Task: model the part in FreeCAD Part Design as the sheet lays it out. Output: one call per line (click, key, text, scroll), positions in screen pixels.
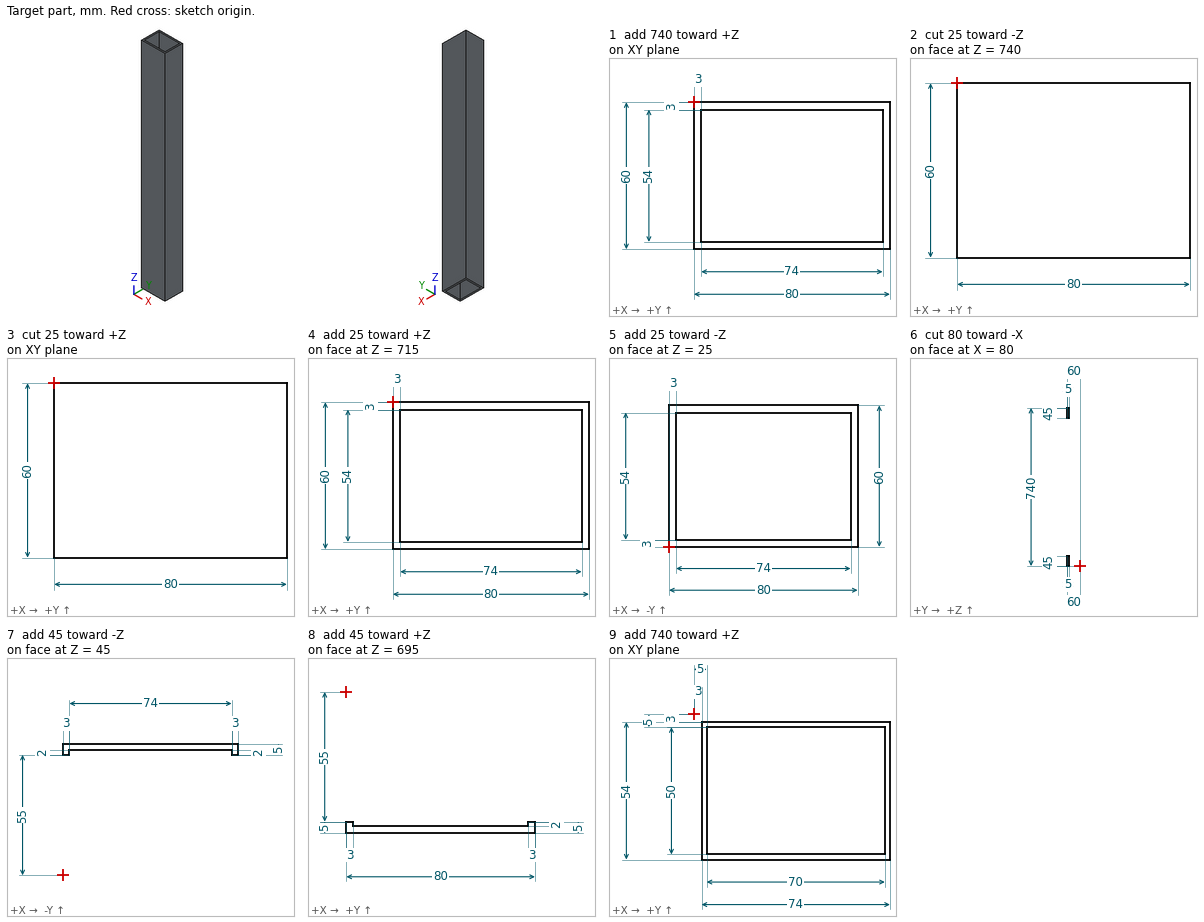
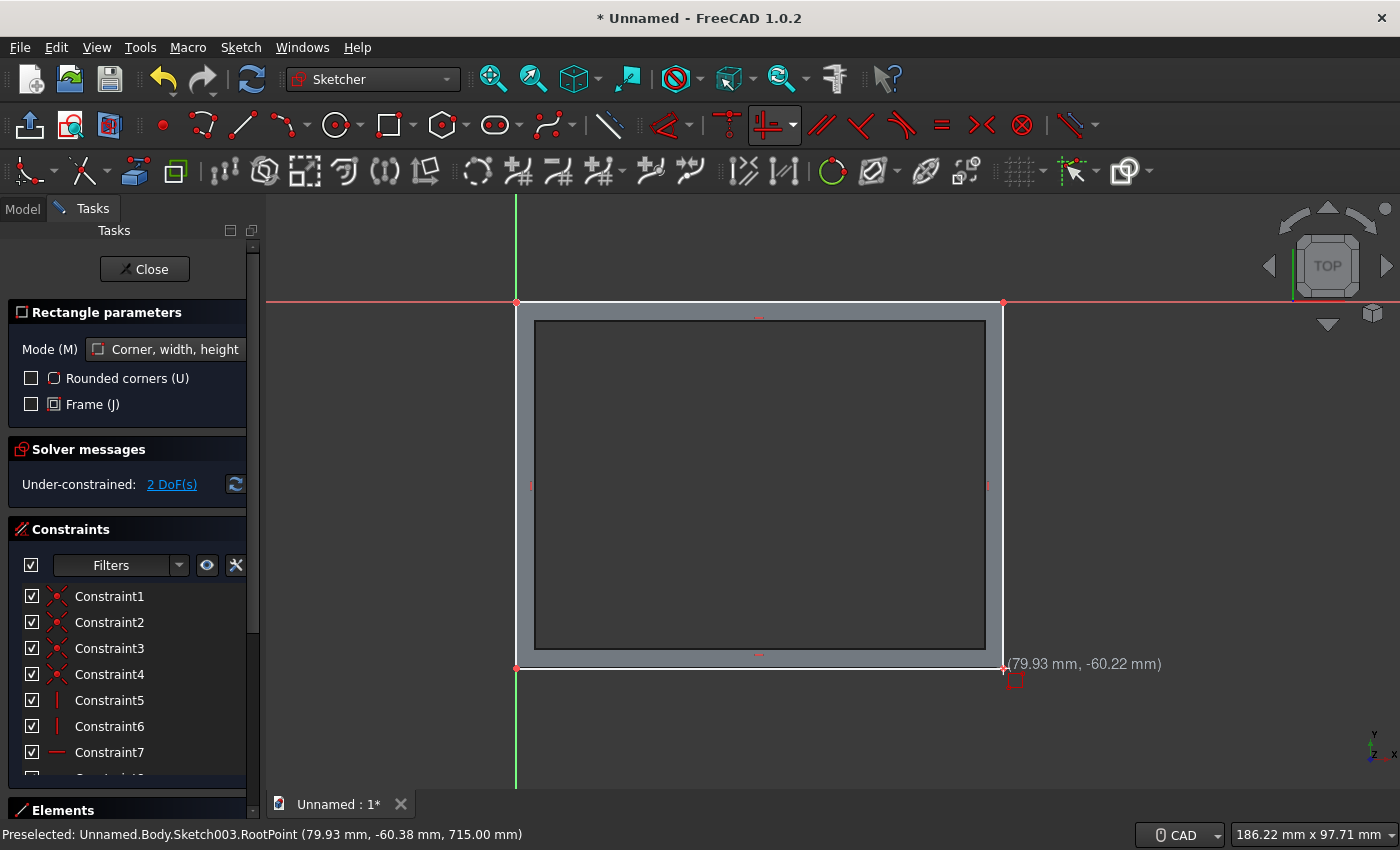
click(535, 321)
click(985, 649)
key(Escape)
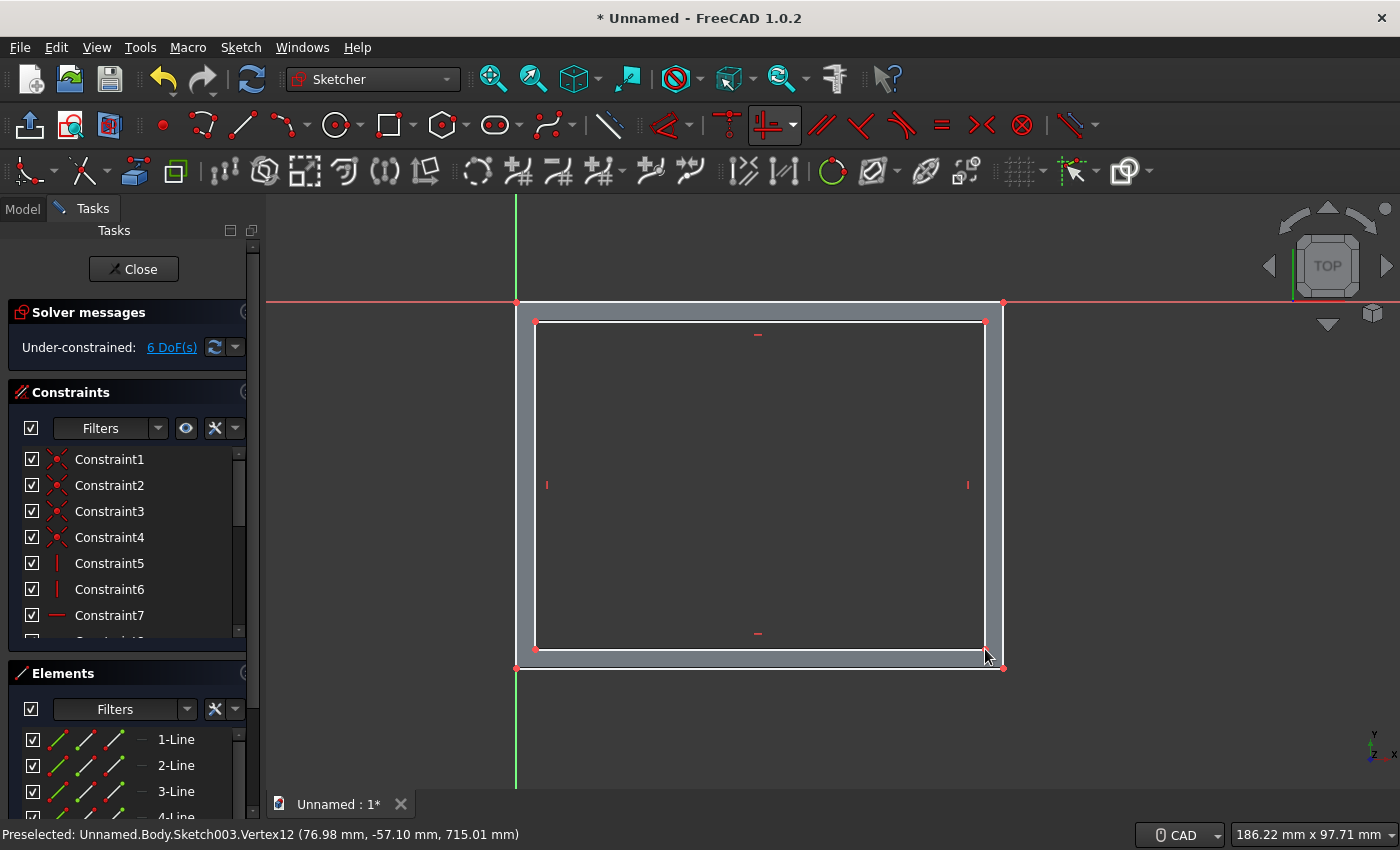
click(664, 126)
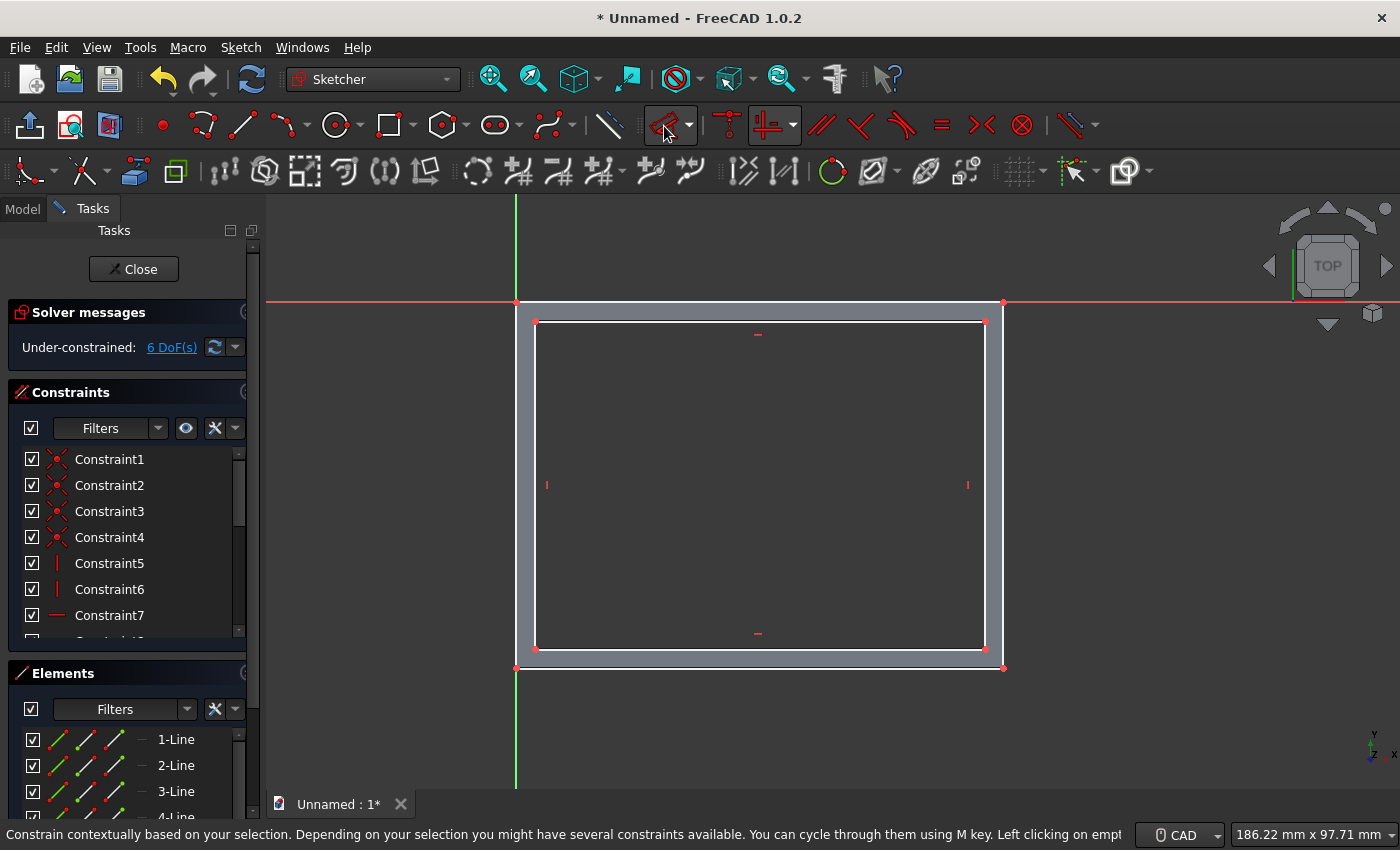
click(516, 412)
click(482, 486)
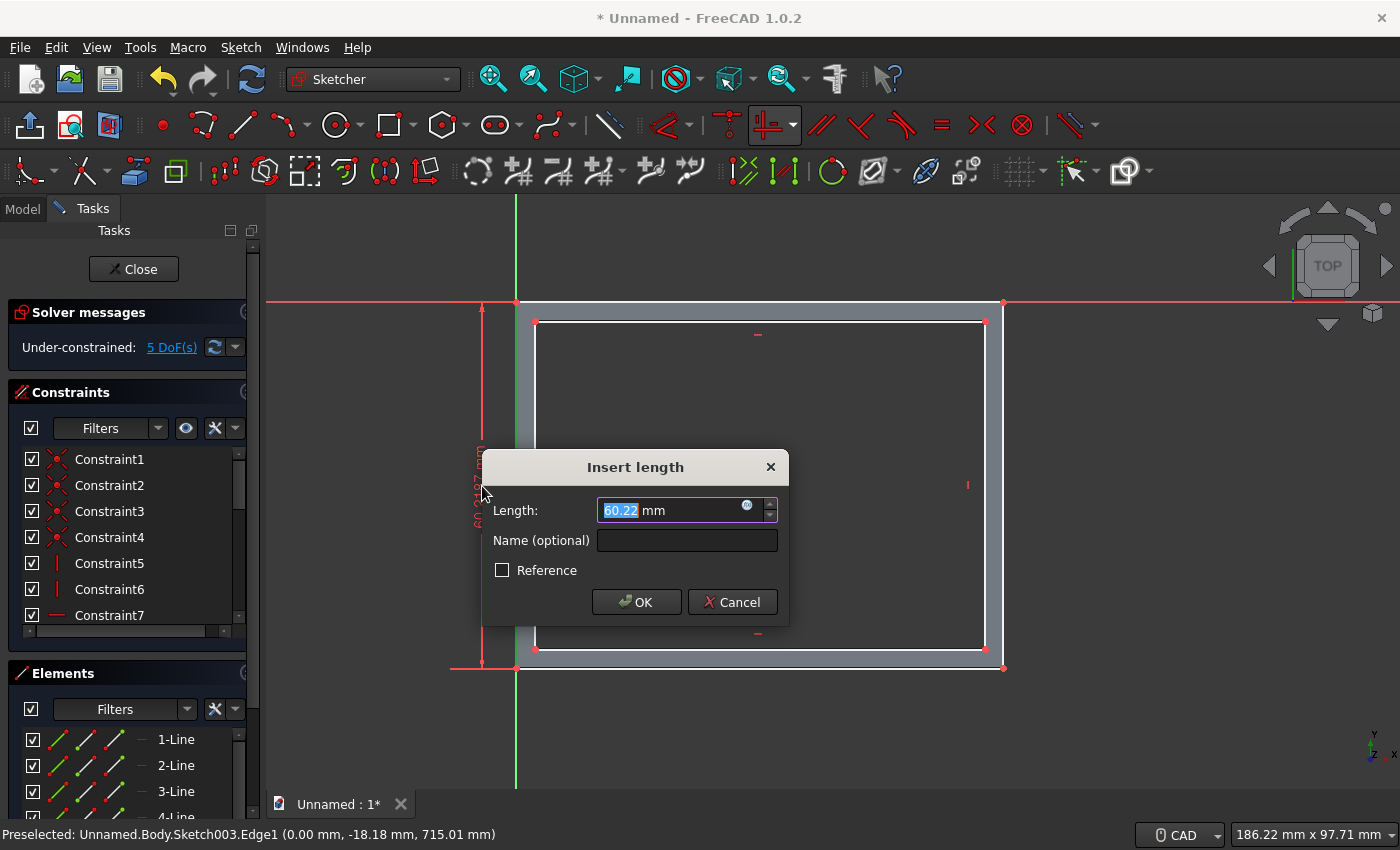
text(60)
key(Return)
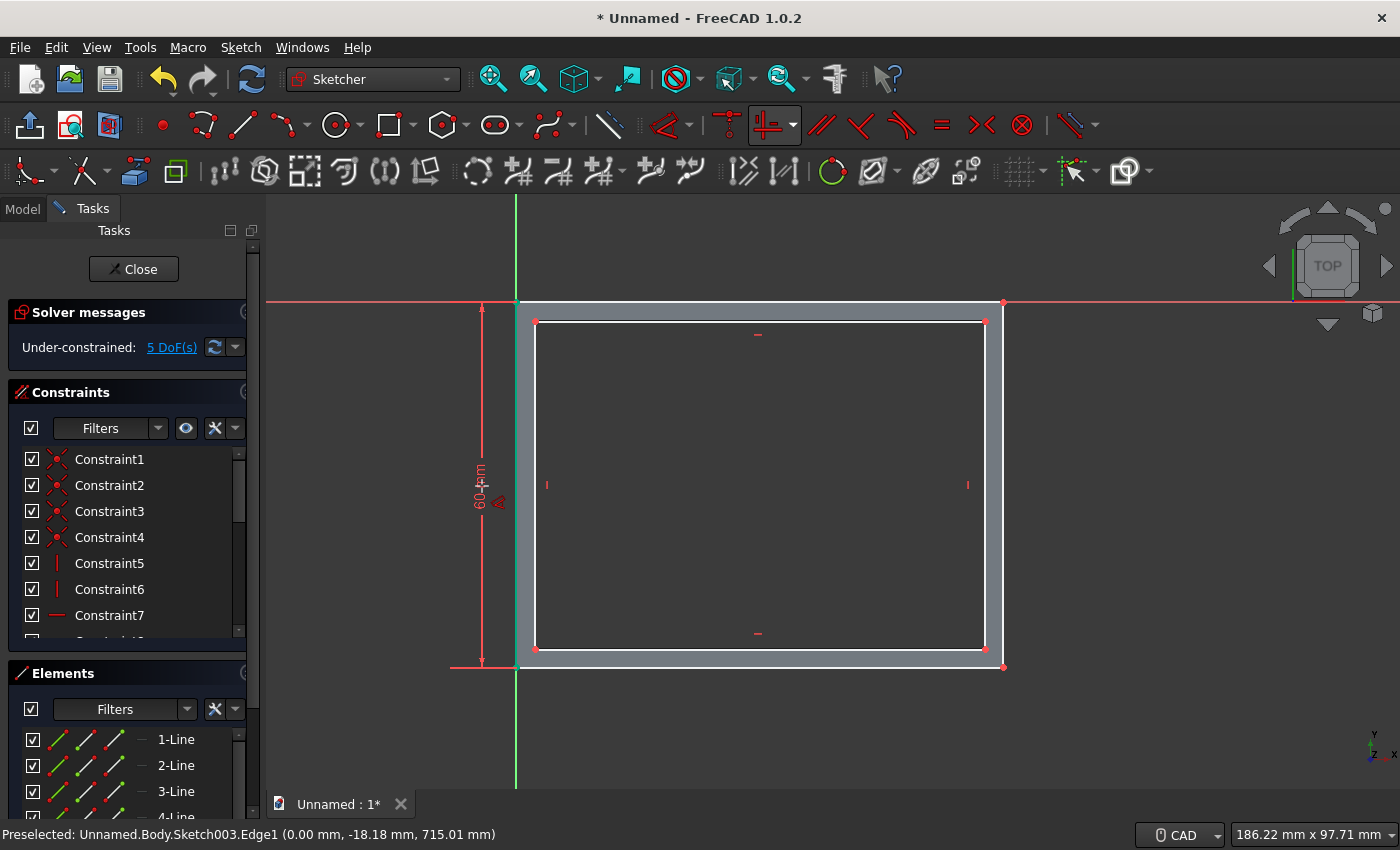
click(662, 668)
click(760, 702)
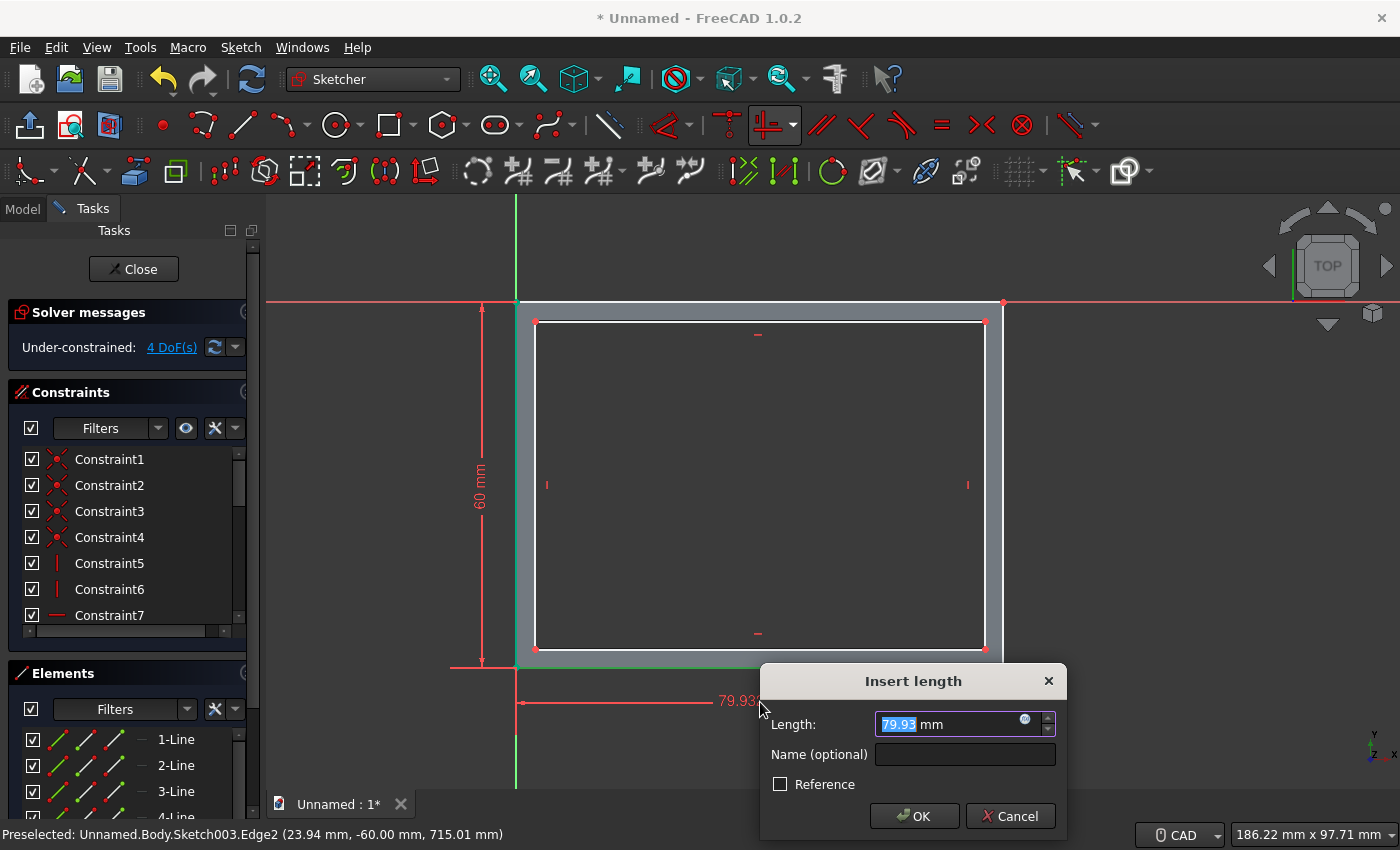
text(80)
key(Return)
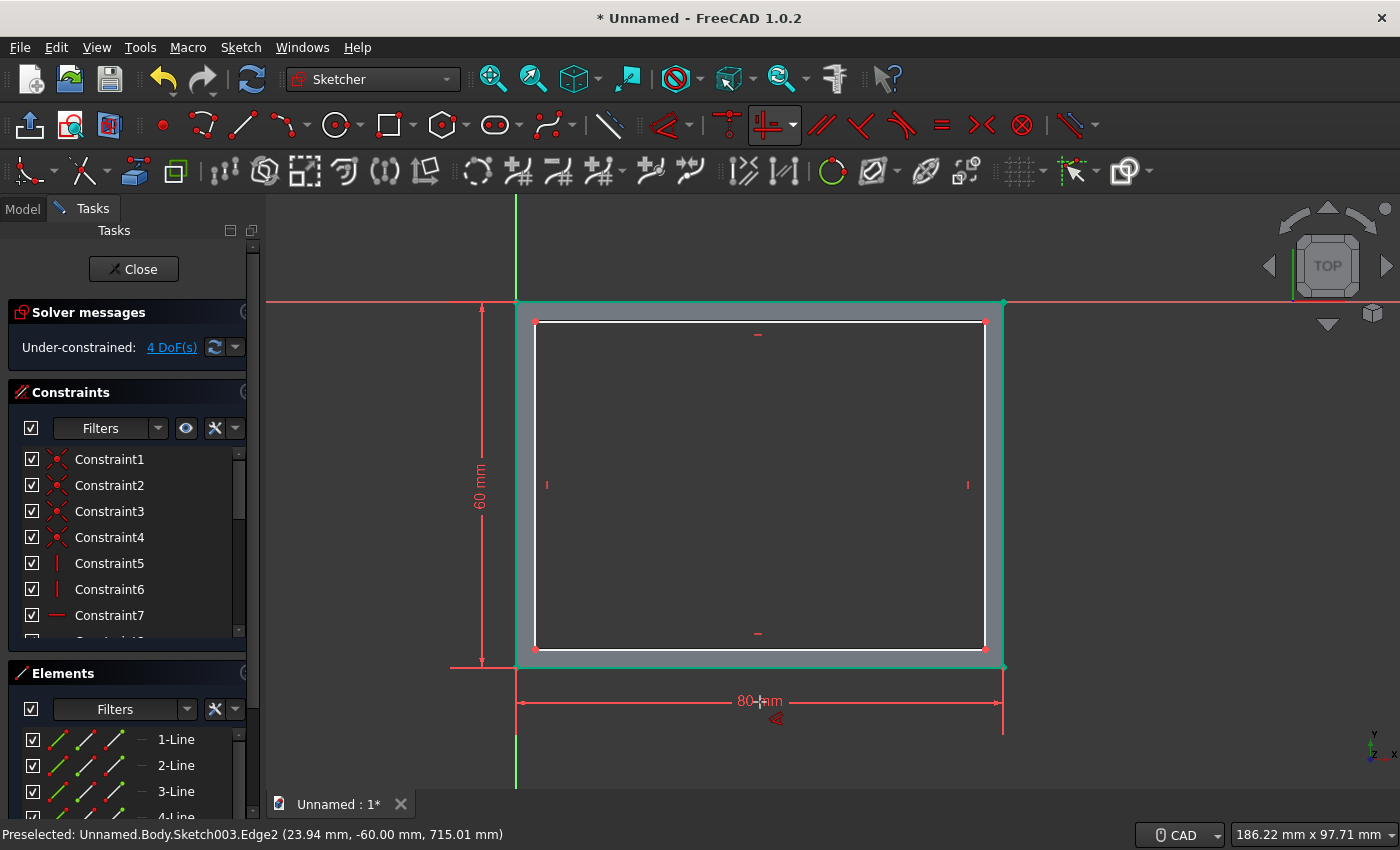
click(535, 420)
click(501, 411)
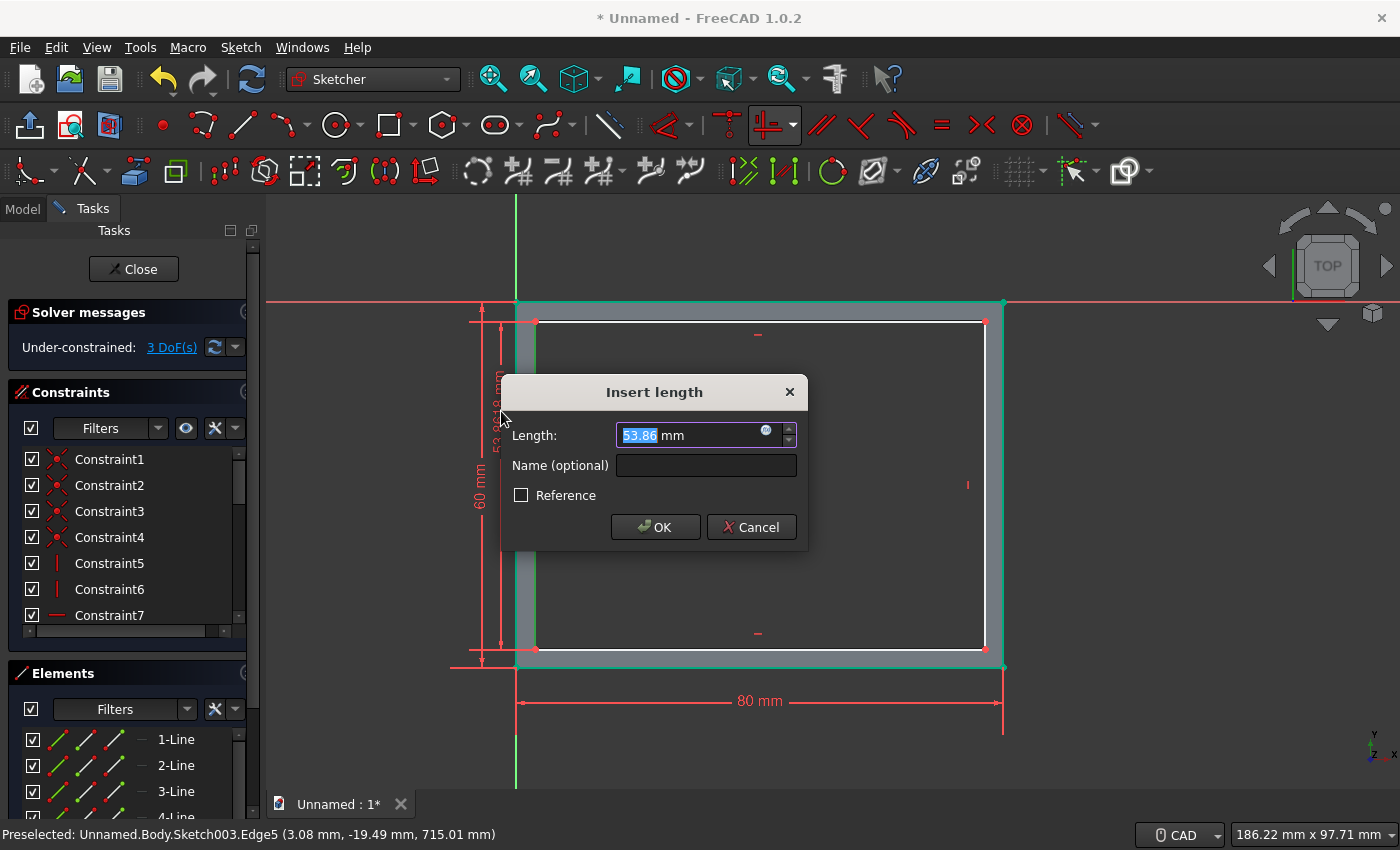
text(54)
key(Return)